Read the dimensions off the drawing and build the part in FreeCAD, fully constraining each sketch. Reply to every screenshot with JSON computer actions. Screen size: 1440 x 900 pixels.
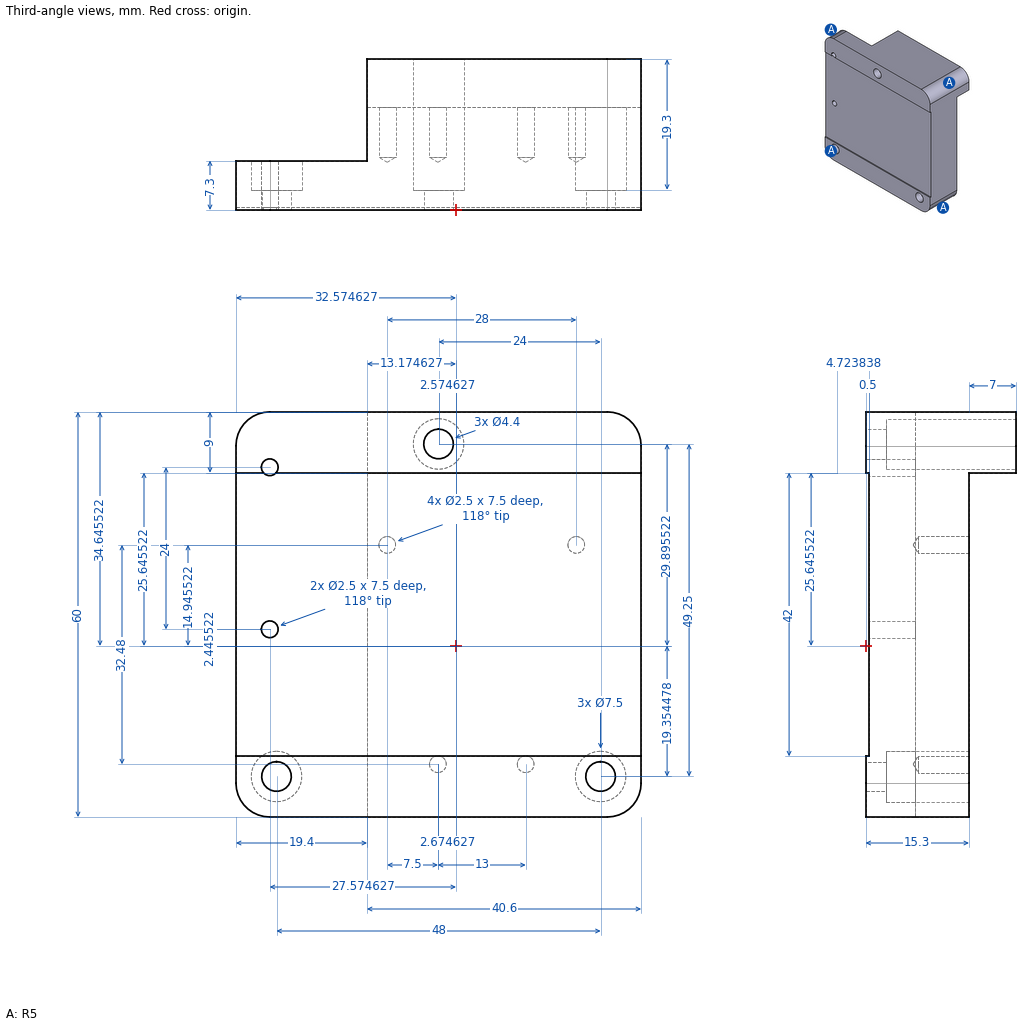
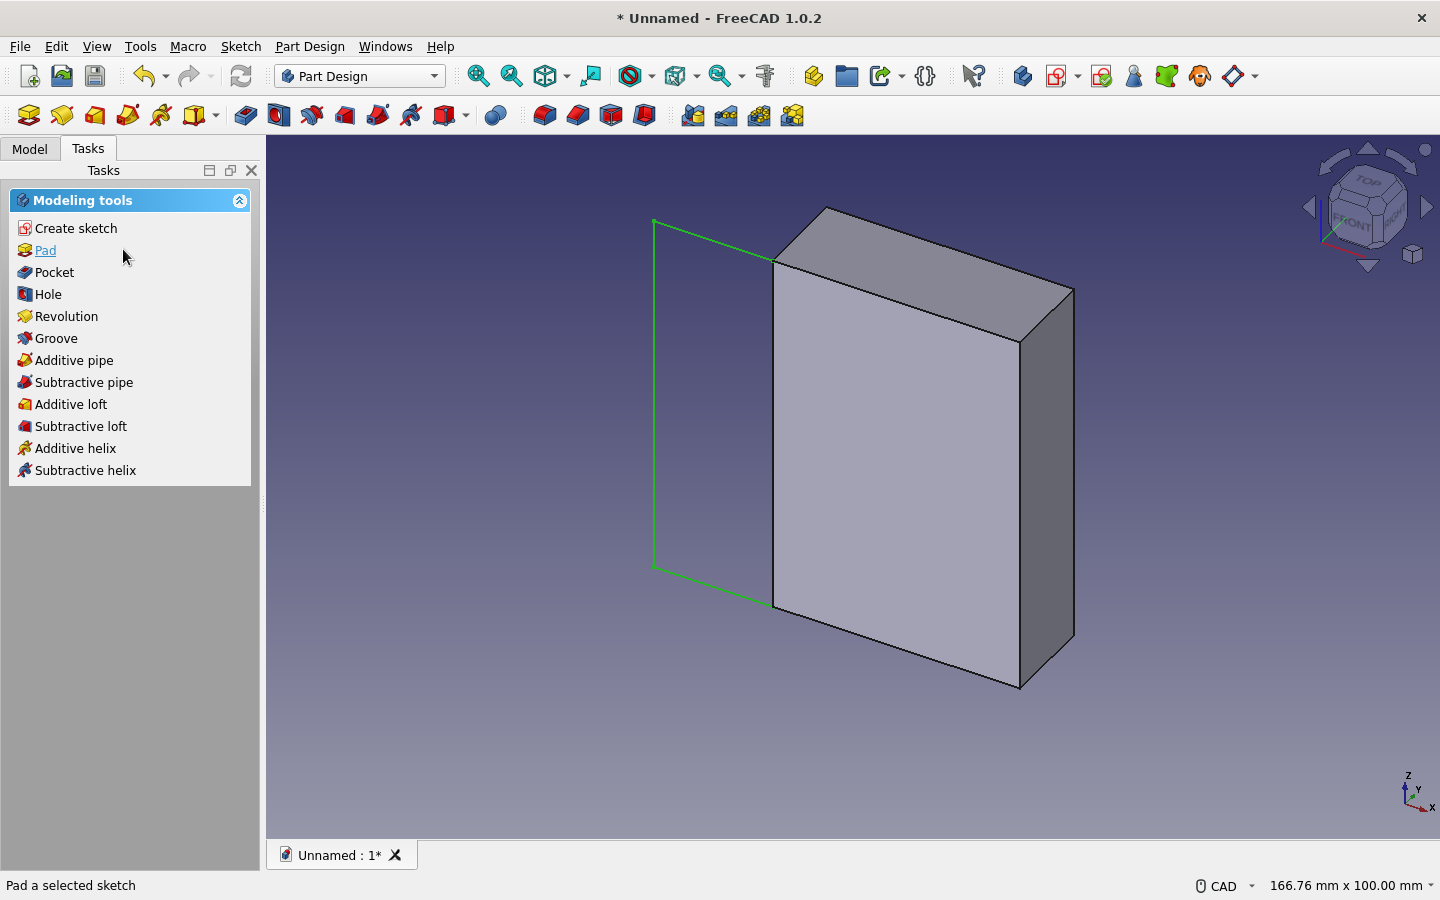
{"action": "left_click", "coordinate": [29, 116]}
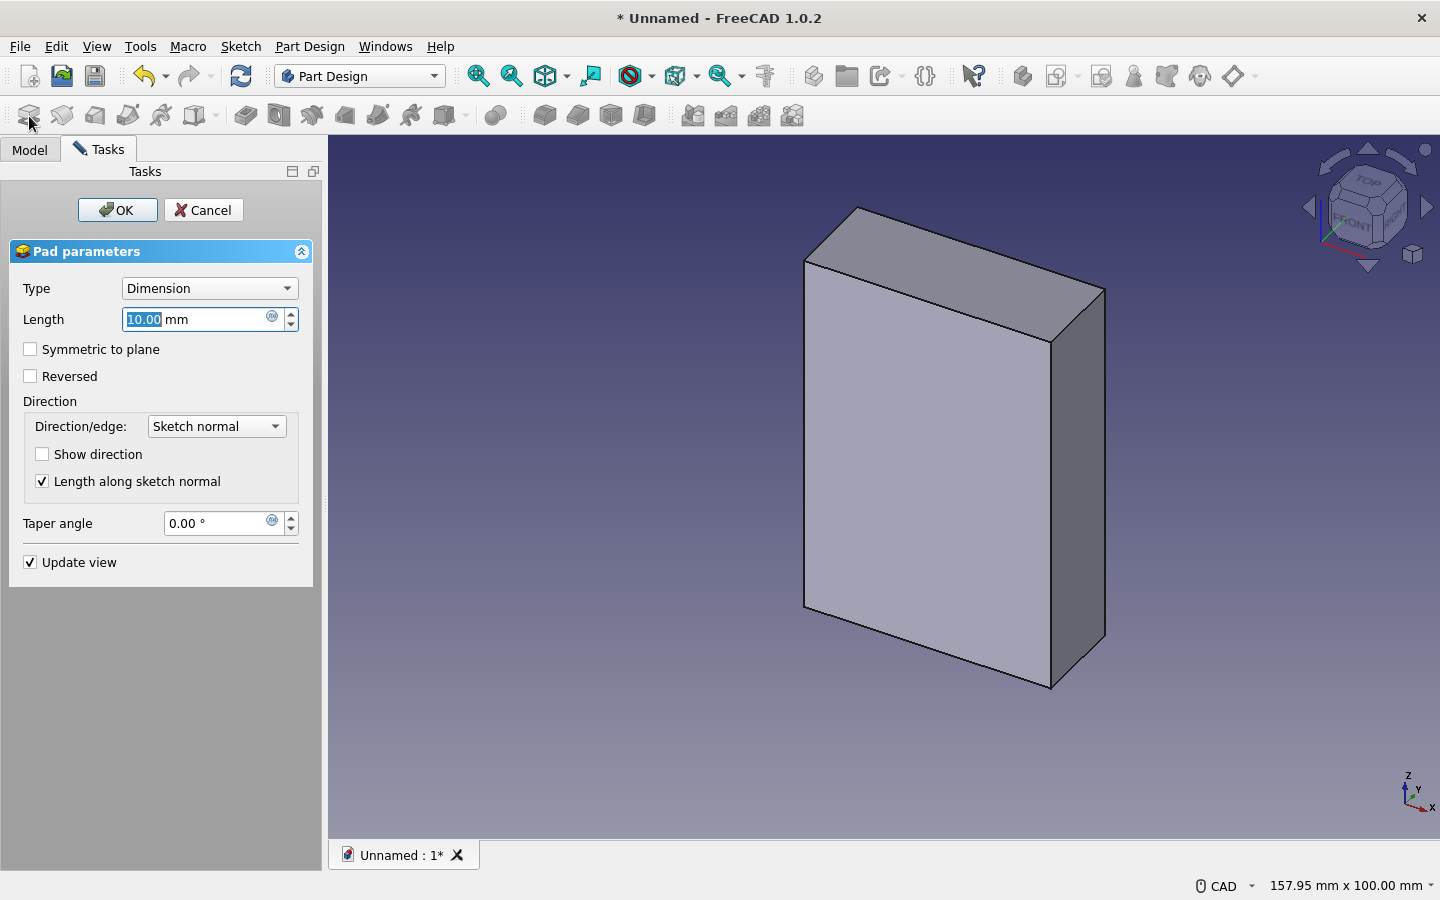
{"action": "type", "text": "7.3"}
{"action": "key", "text": "Tab"}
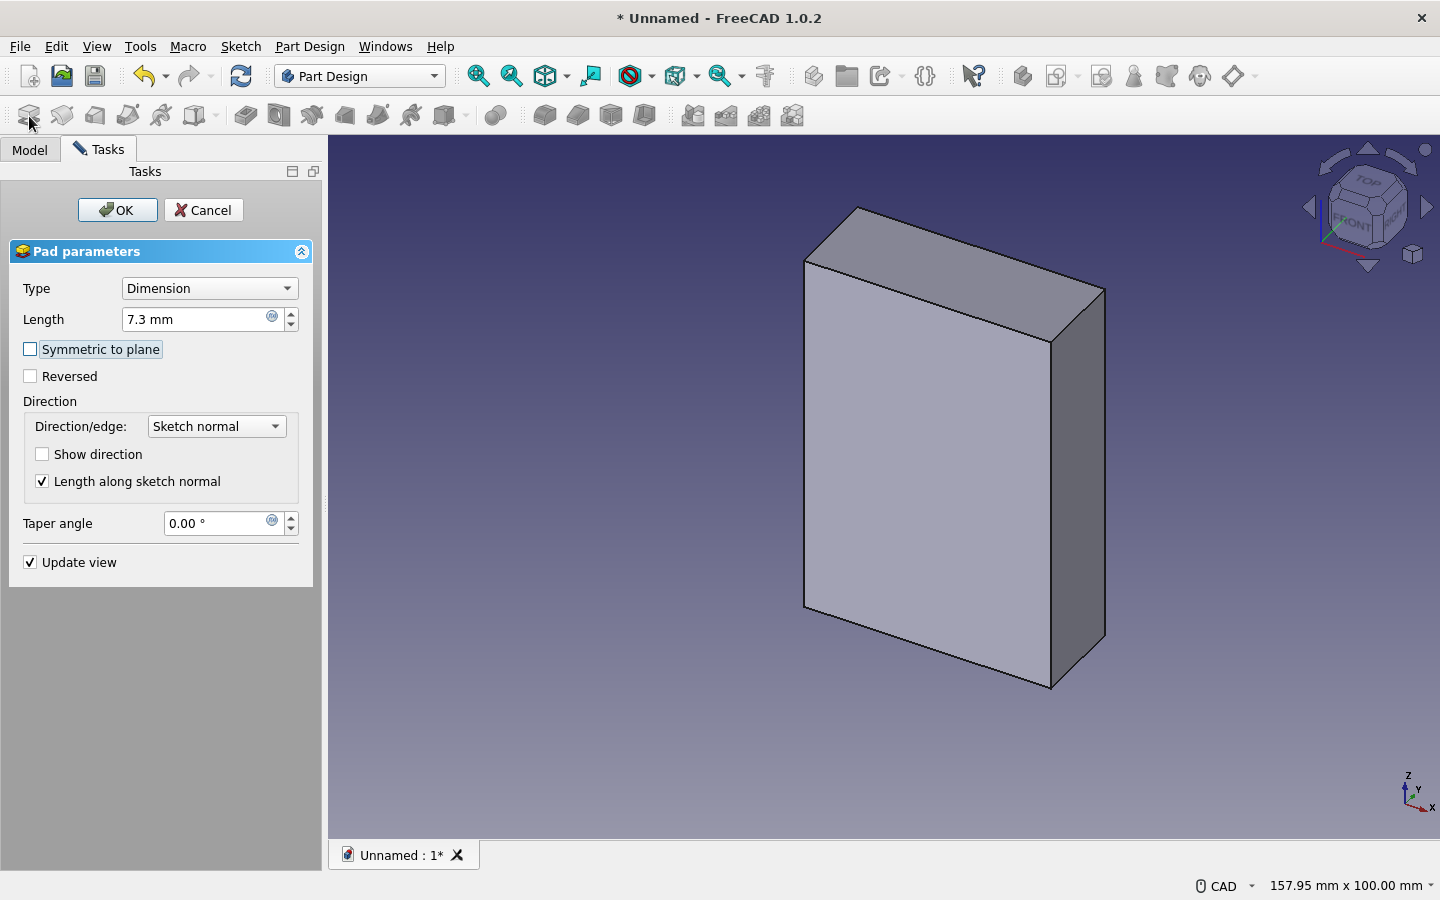
{"action": "left_click", "coordinate": [31, 376]}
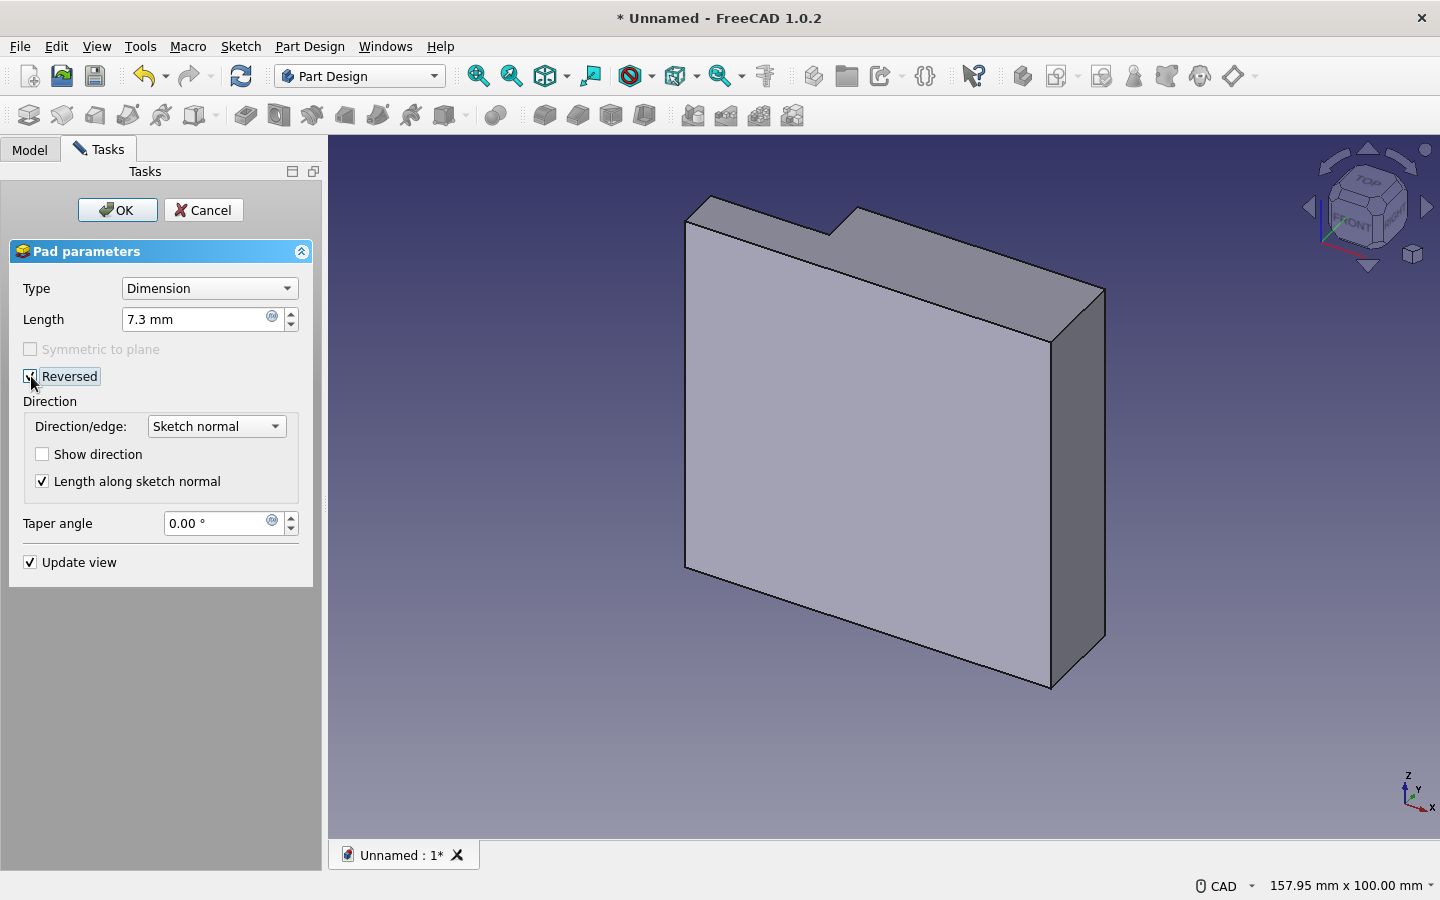
{"action": "left_click", "coordinate": [118, 210]}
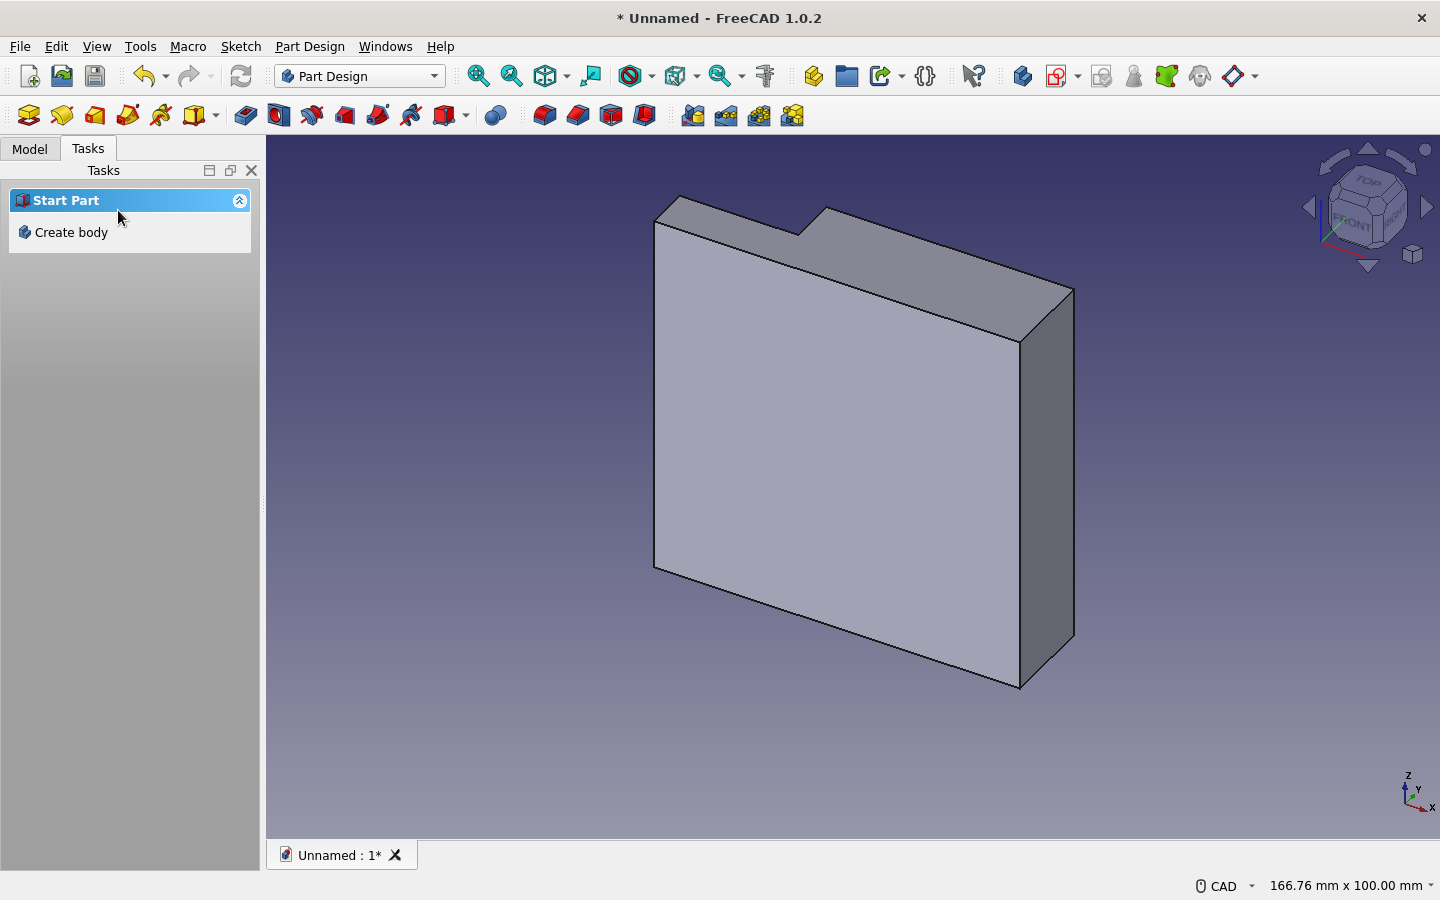
{"action": "key", "text": "4"}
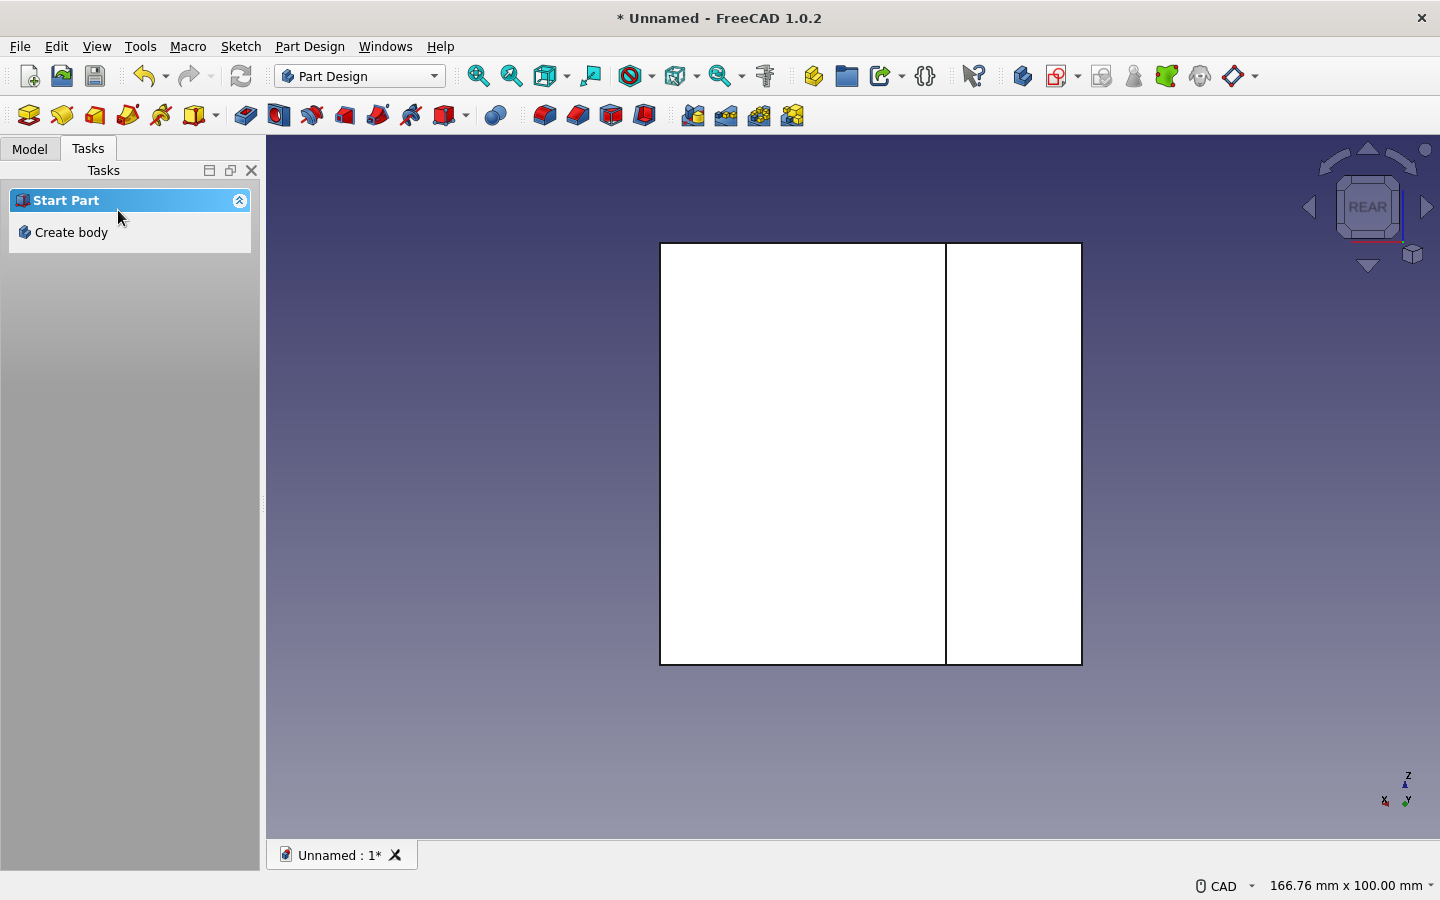
{"action": "left_click", "coordinate": [803, 393]}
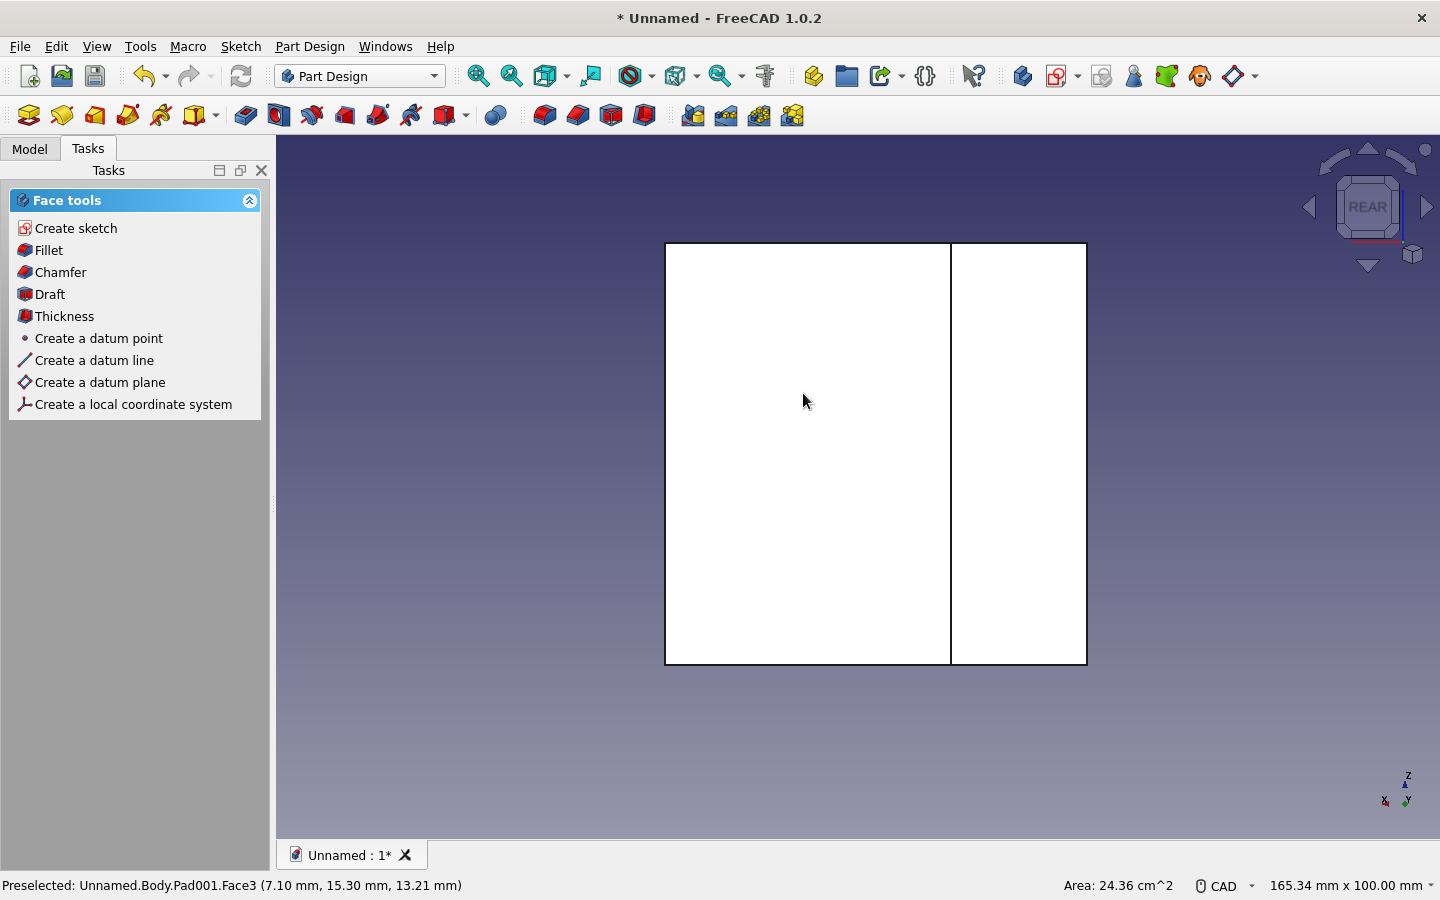
{"action": "left_click", "coordinate": [1056, 76]}